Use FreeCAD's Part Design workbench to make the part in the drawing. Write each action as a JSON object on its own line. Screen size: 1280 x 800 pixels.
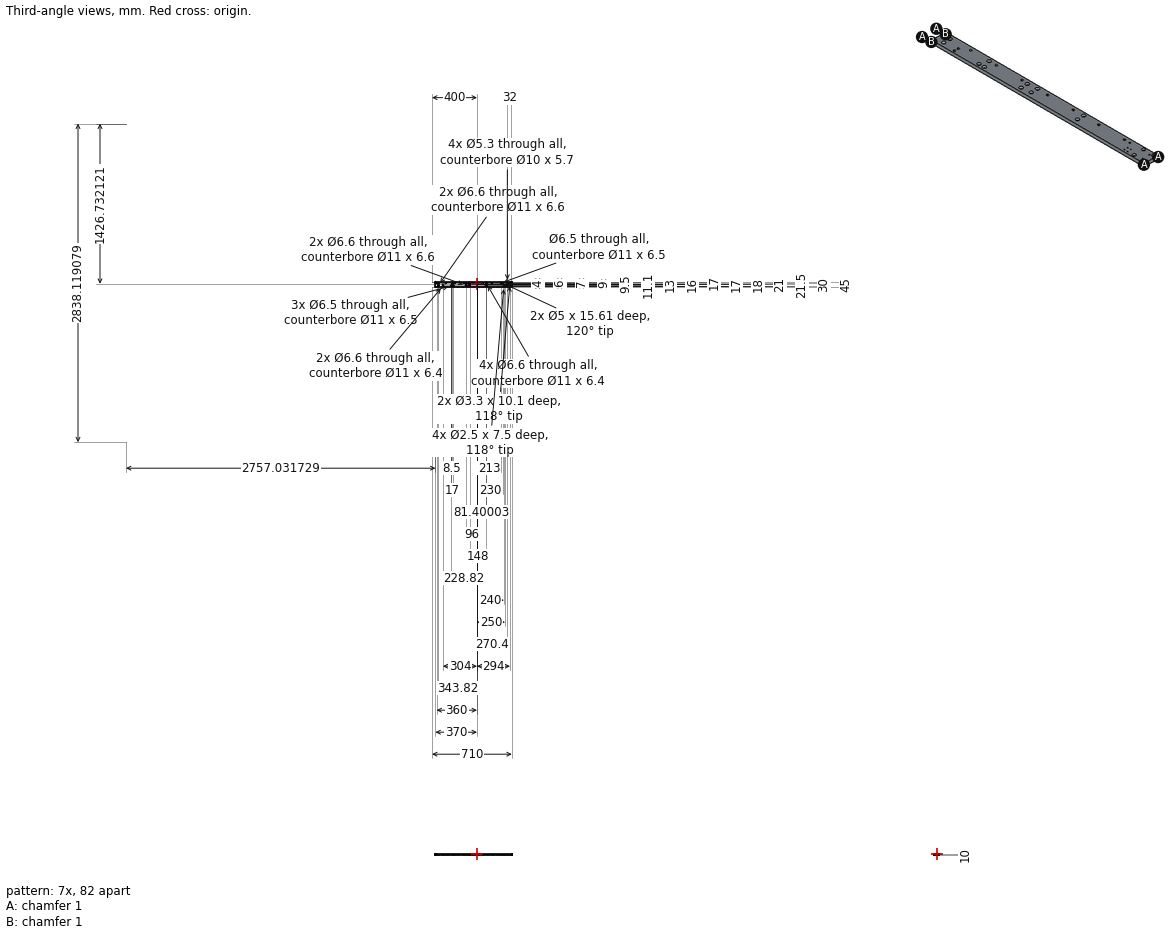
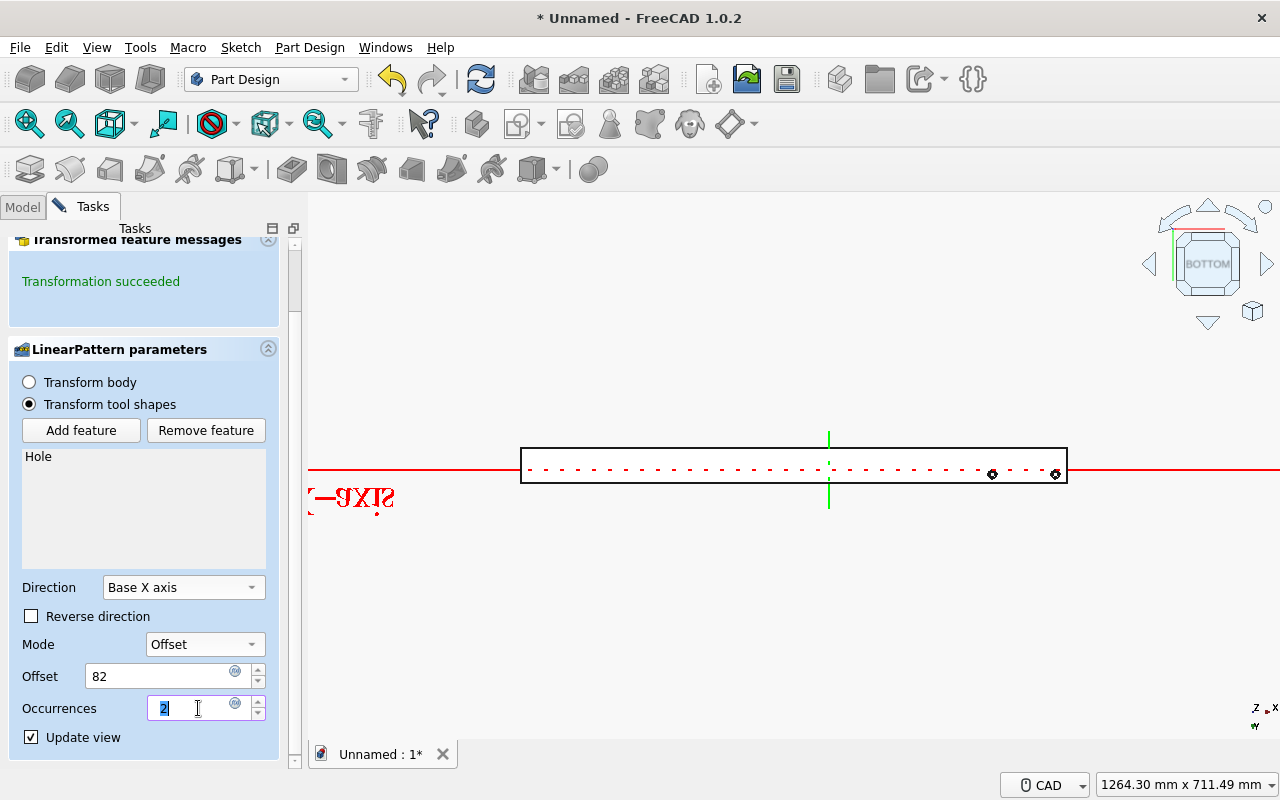
{"action": "type", "text": "7"}
{"action": "key", "text": "Tab"}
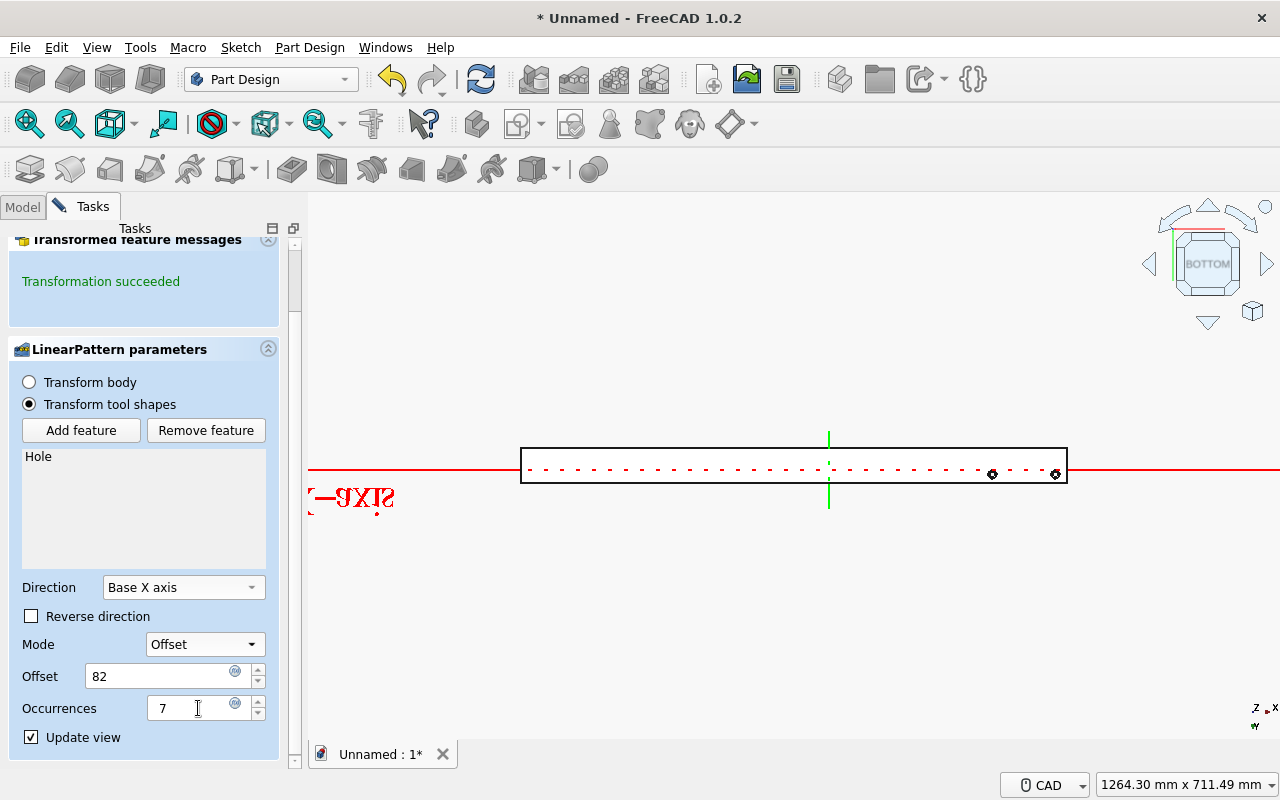
{"action": "left_click", "coordinate": [30, 616]}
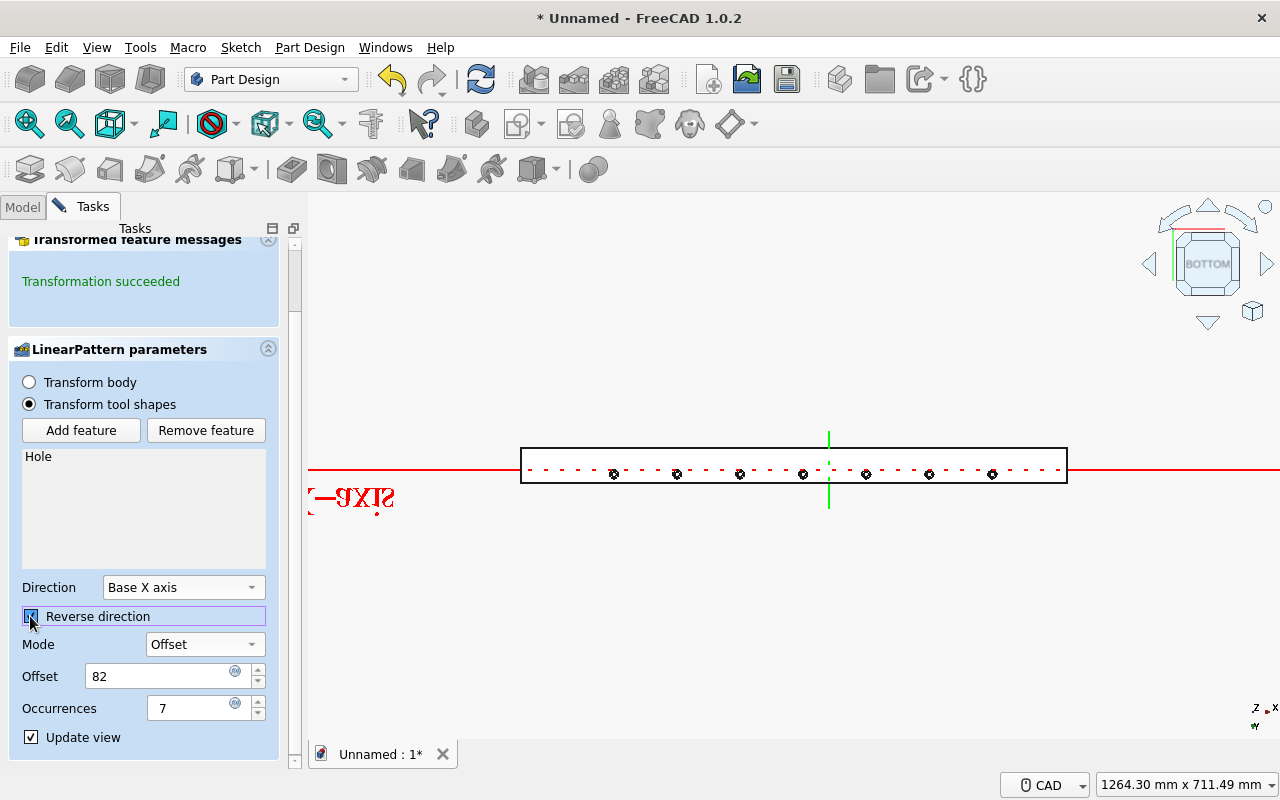
{"action": "scroll", "coordinate": [295, 503], "scroll_direction": "up", "scroll_amount": 2}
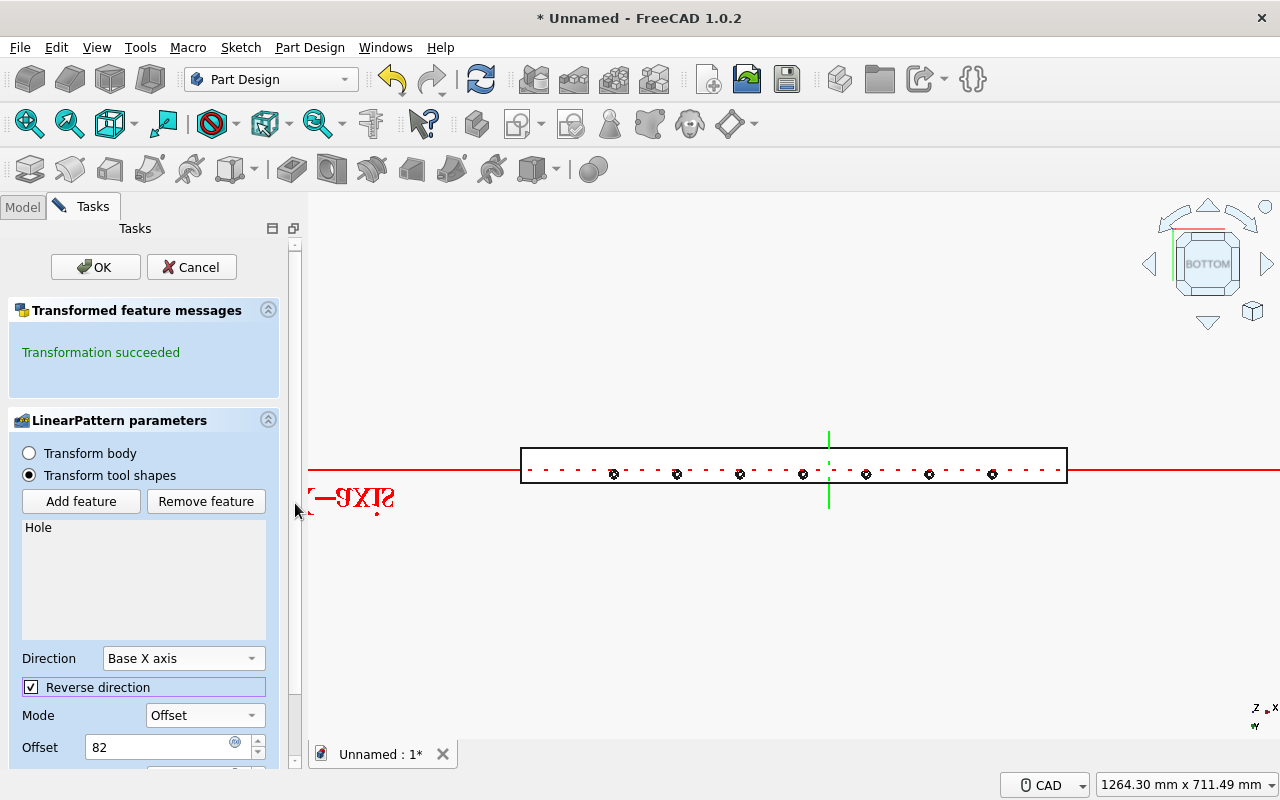
{"action": "left_click", "coordinate": [96, 267]}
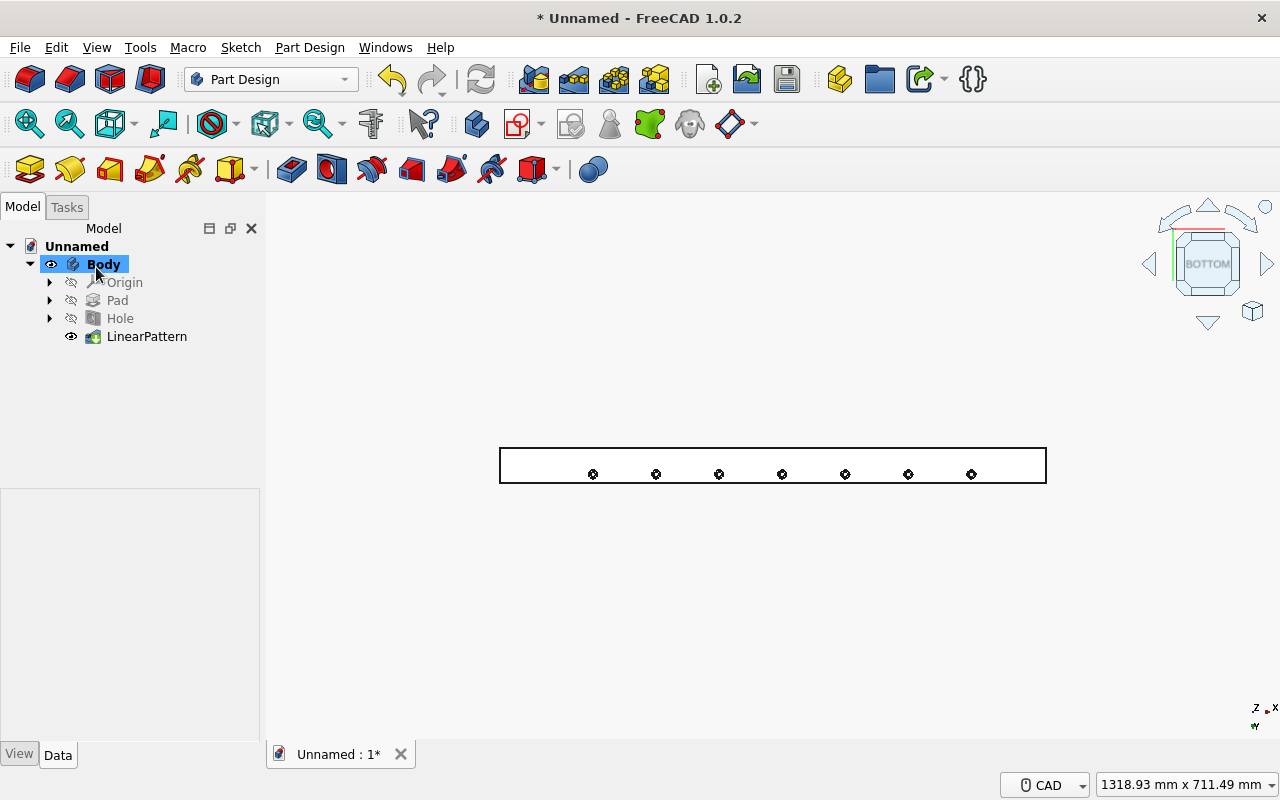
{"action": "left_click", "coordinate": [518, 124]}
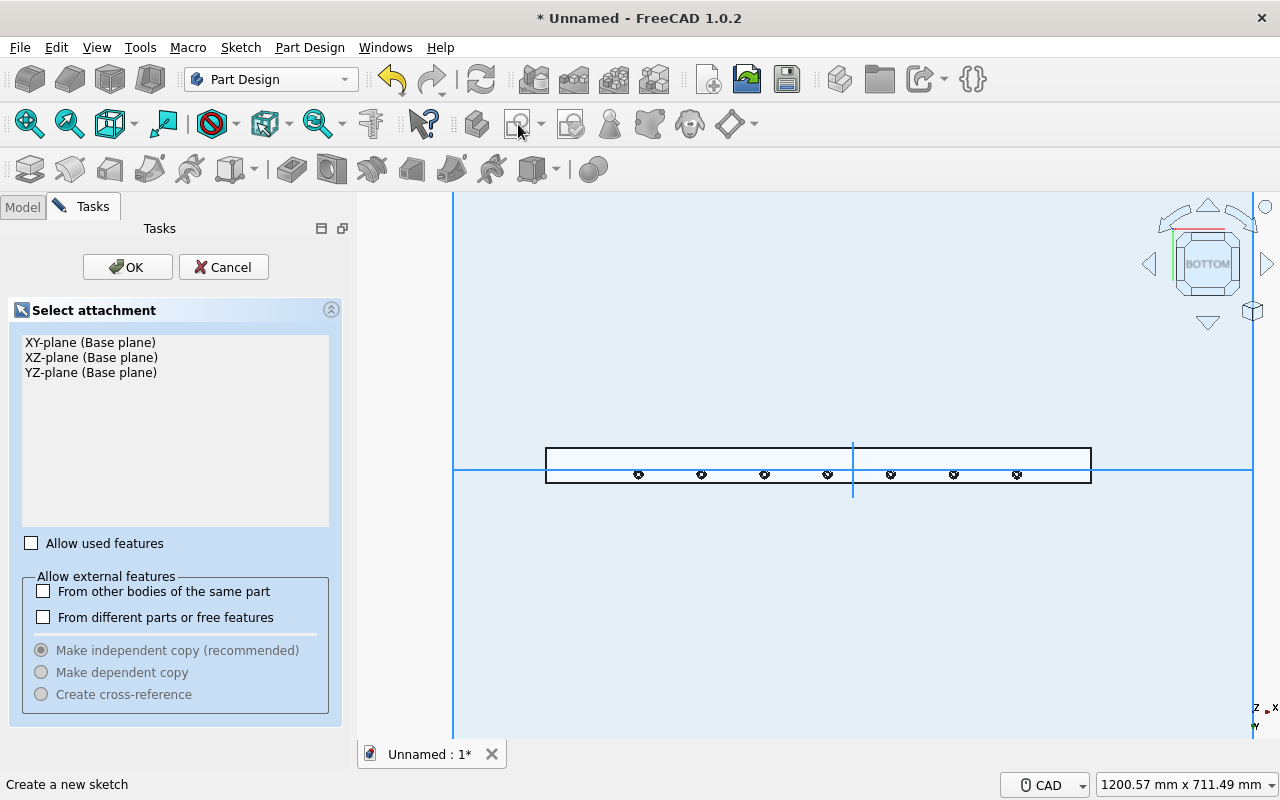
{"action": "left_click", "coordinate": [82, 342]}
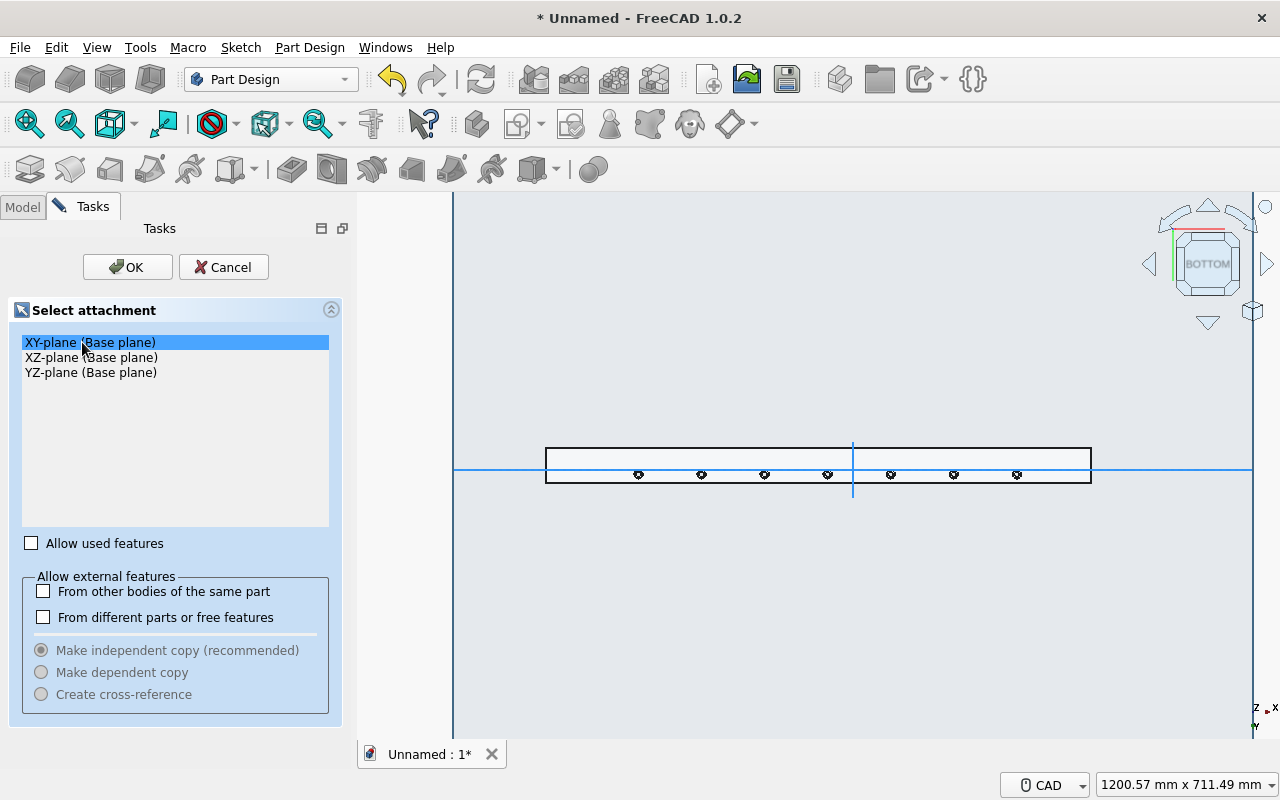
{"action": "left_click", "coordinate": [128, 267]}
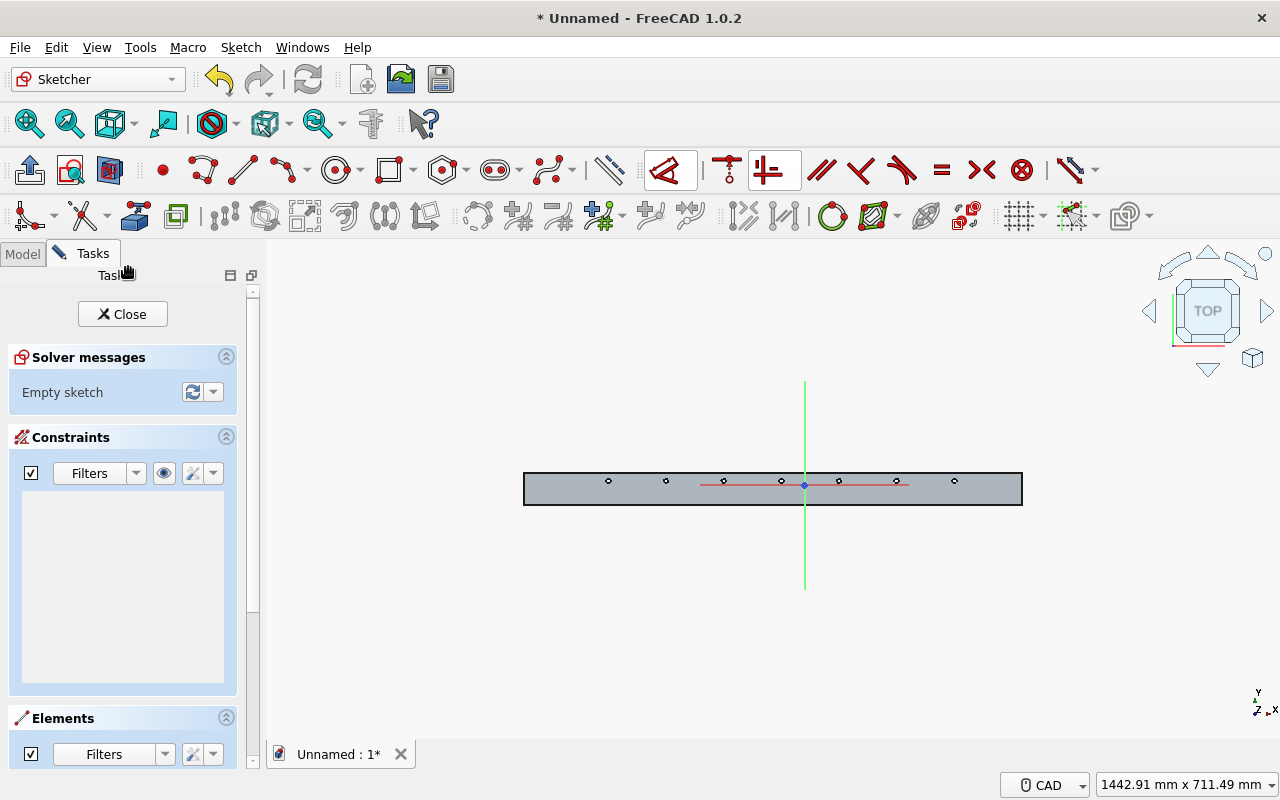
{"action": "scroll", "coordinate": [554, 489], "scroll_direction": "up", "scroll_amount": 14}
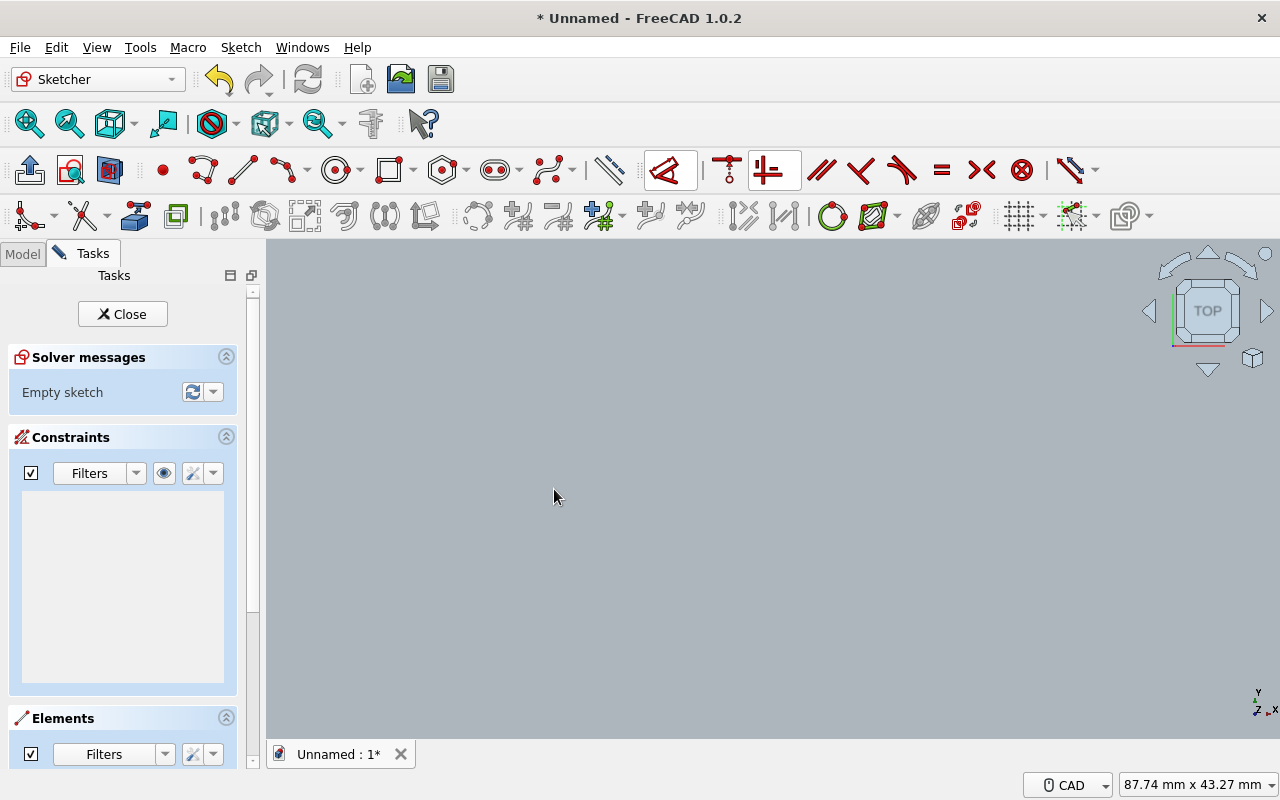
{"action": "left_click", "coordinate": [336, 170]}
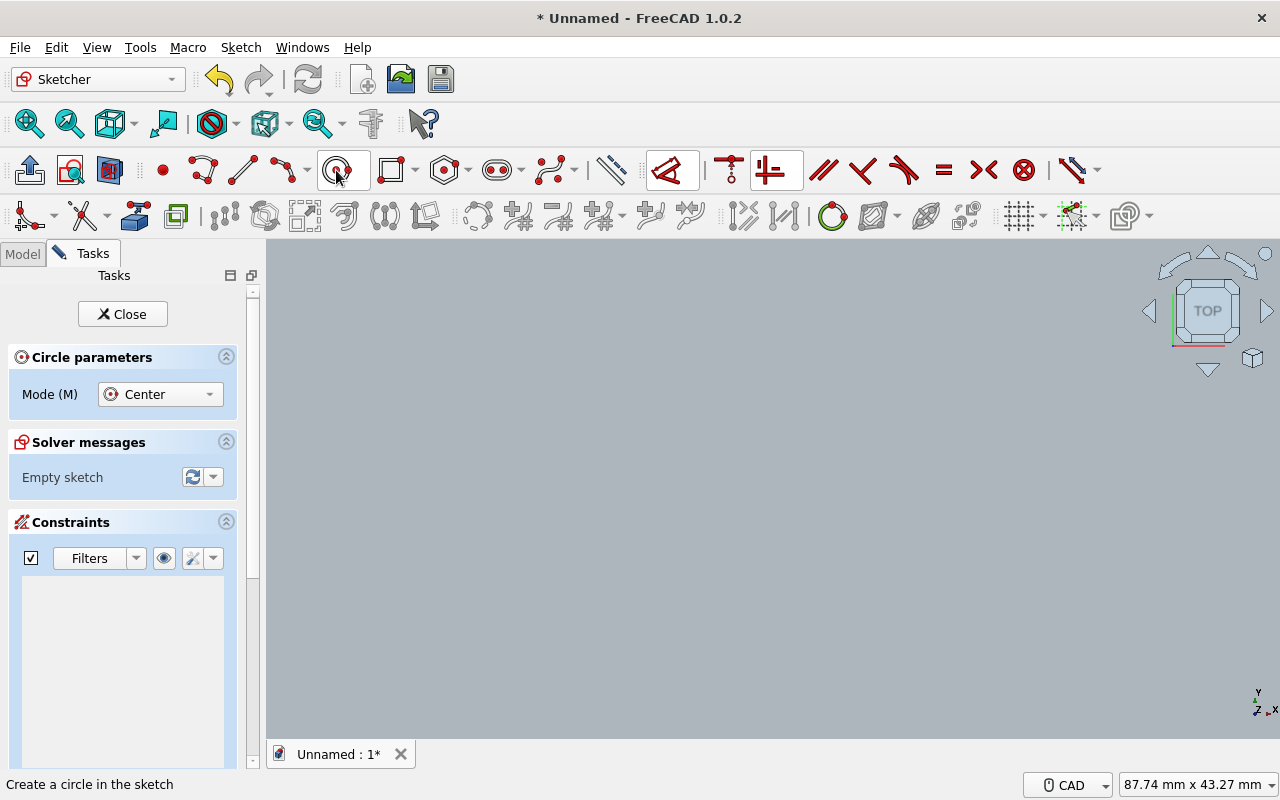
{"action": "left_click", "coordinate": [698, 603]}
{"action": "left_click", "coordinate": [725, 576]}